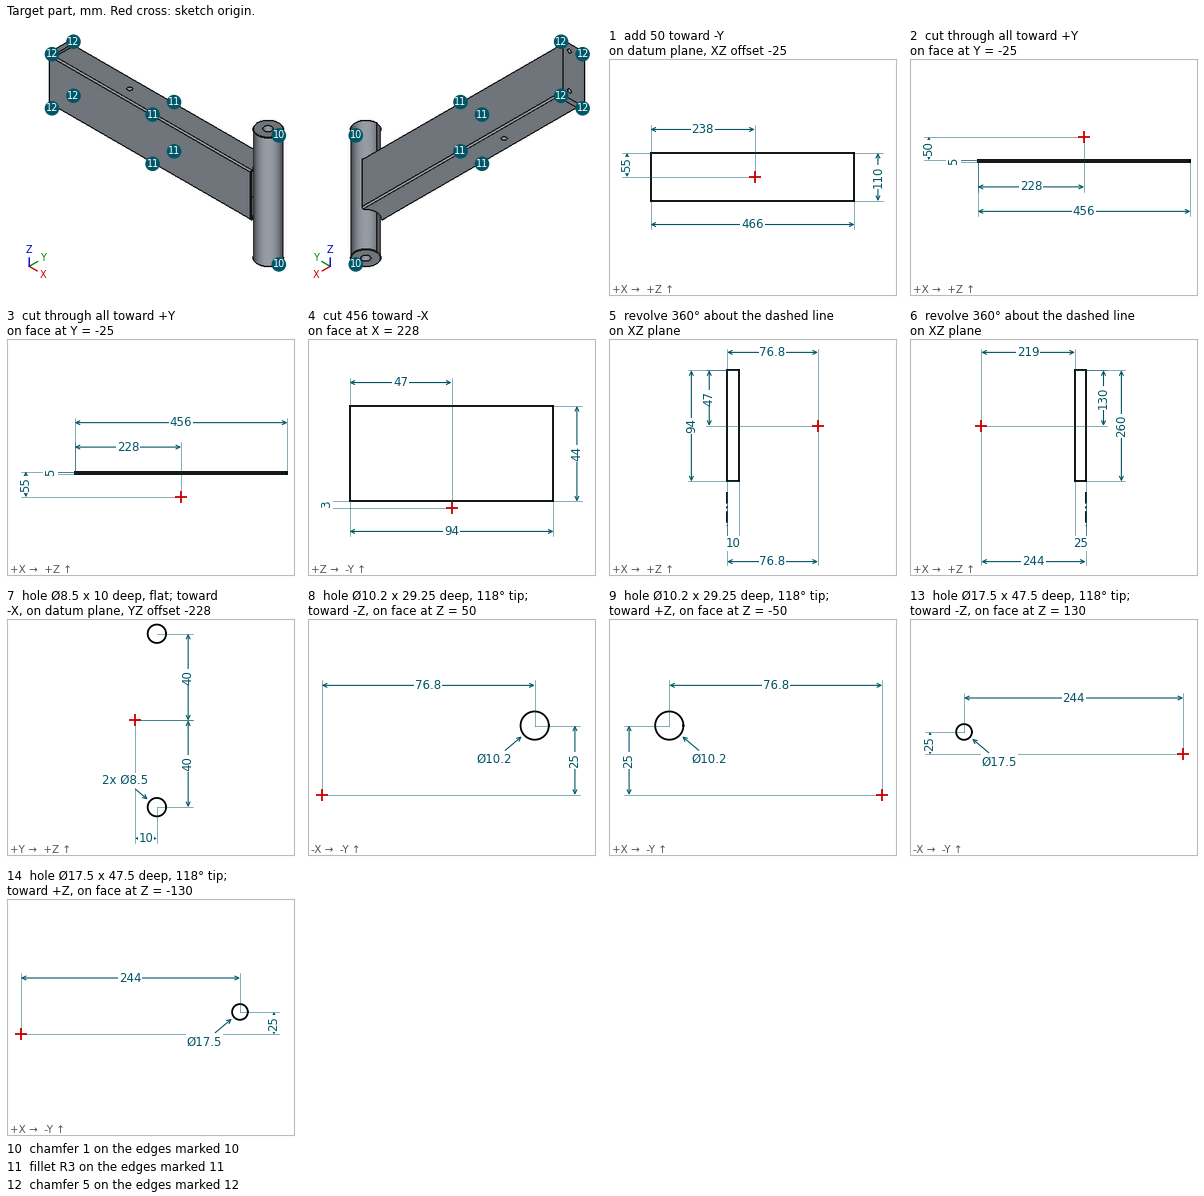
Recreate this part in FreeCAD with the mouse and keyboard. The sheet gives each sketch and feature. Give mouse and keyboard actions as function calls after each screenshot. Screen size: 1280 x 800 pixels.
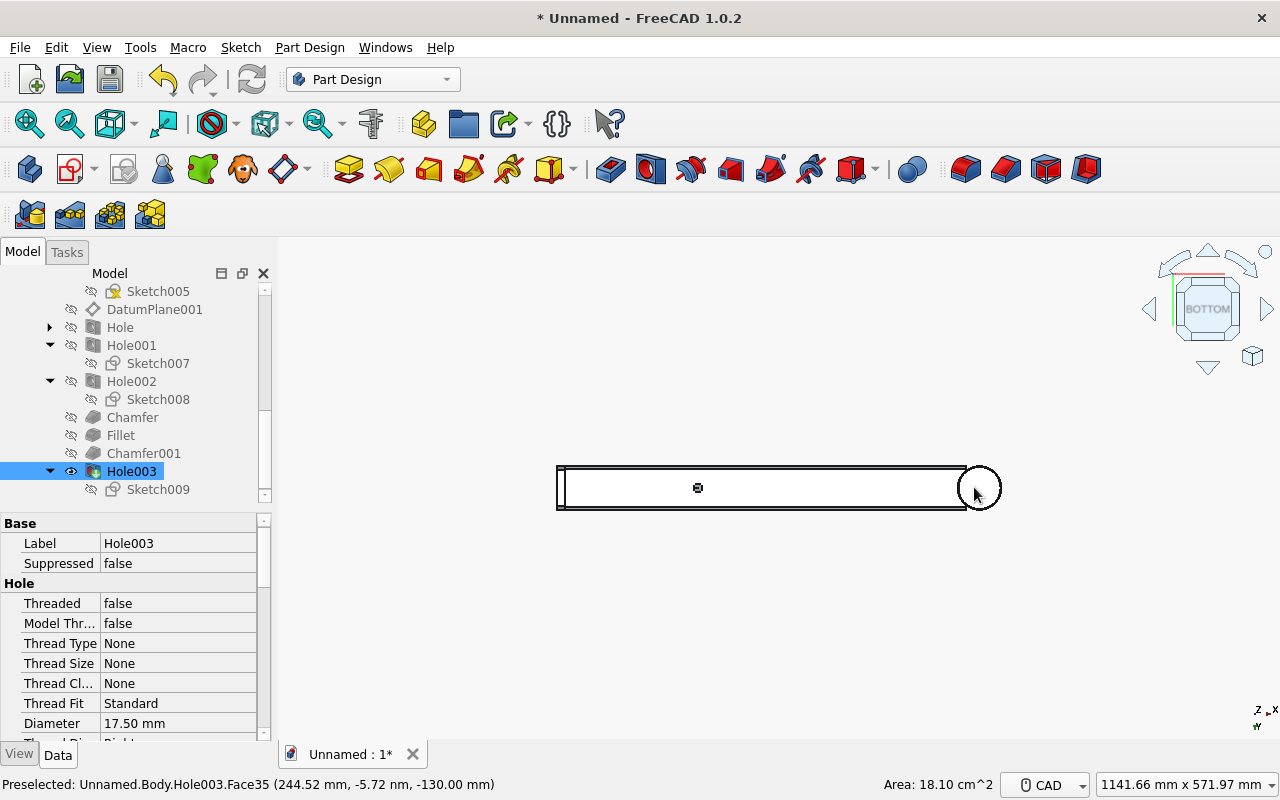
click(70, 170)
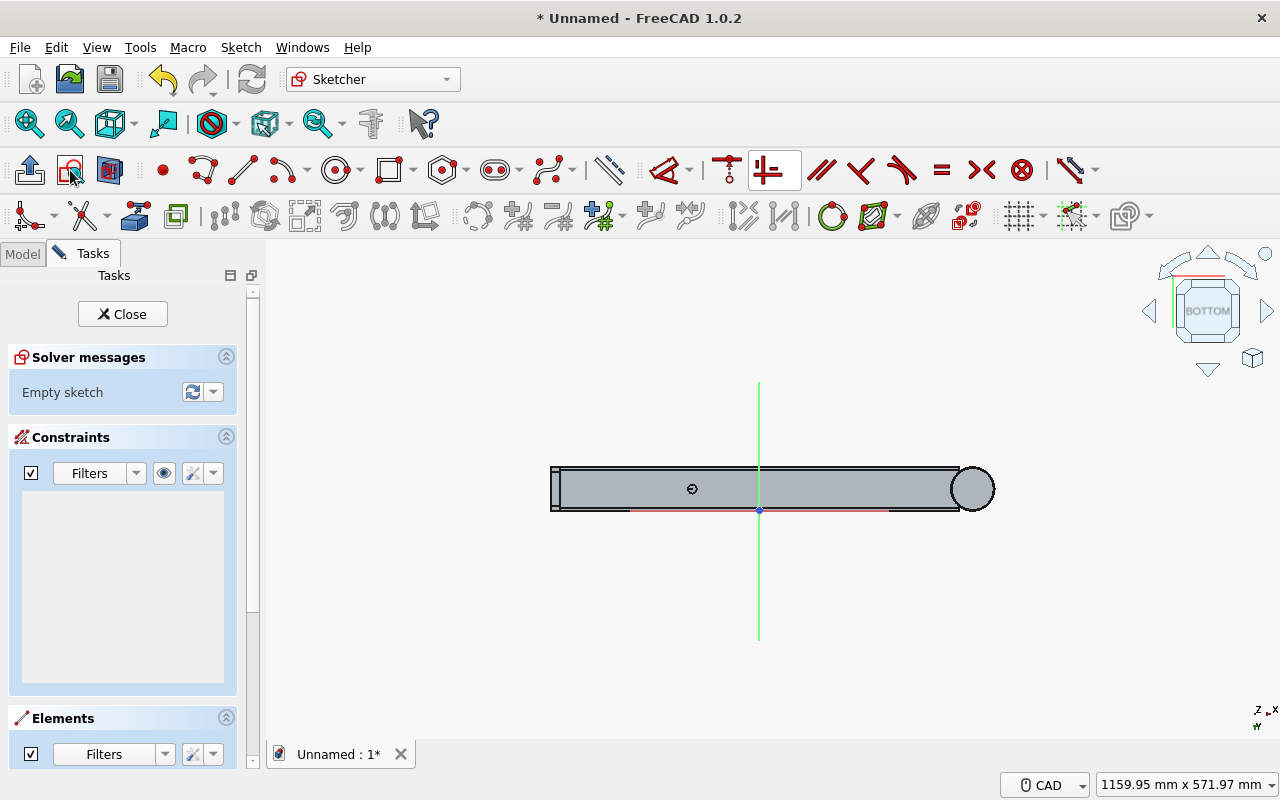
scroll(987, 489, up, 15)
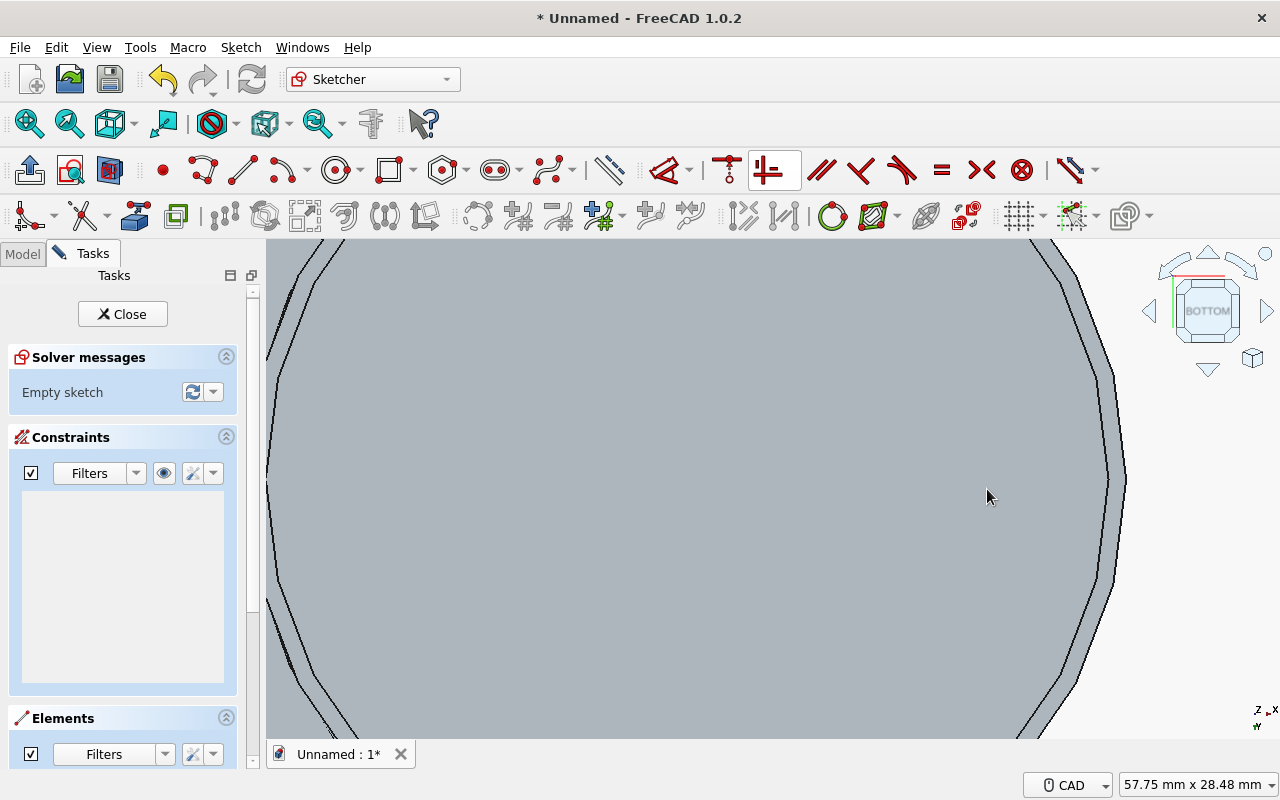
click(336, 170)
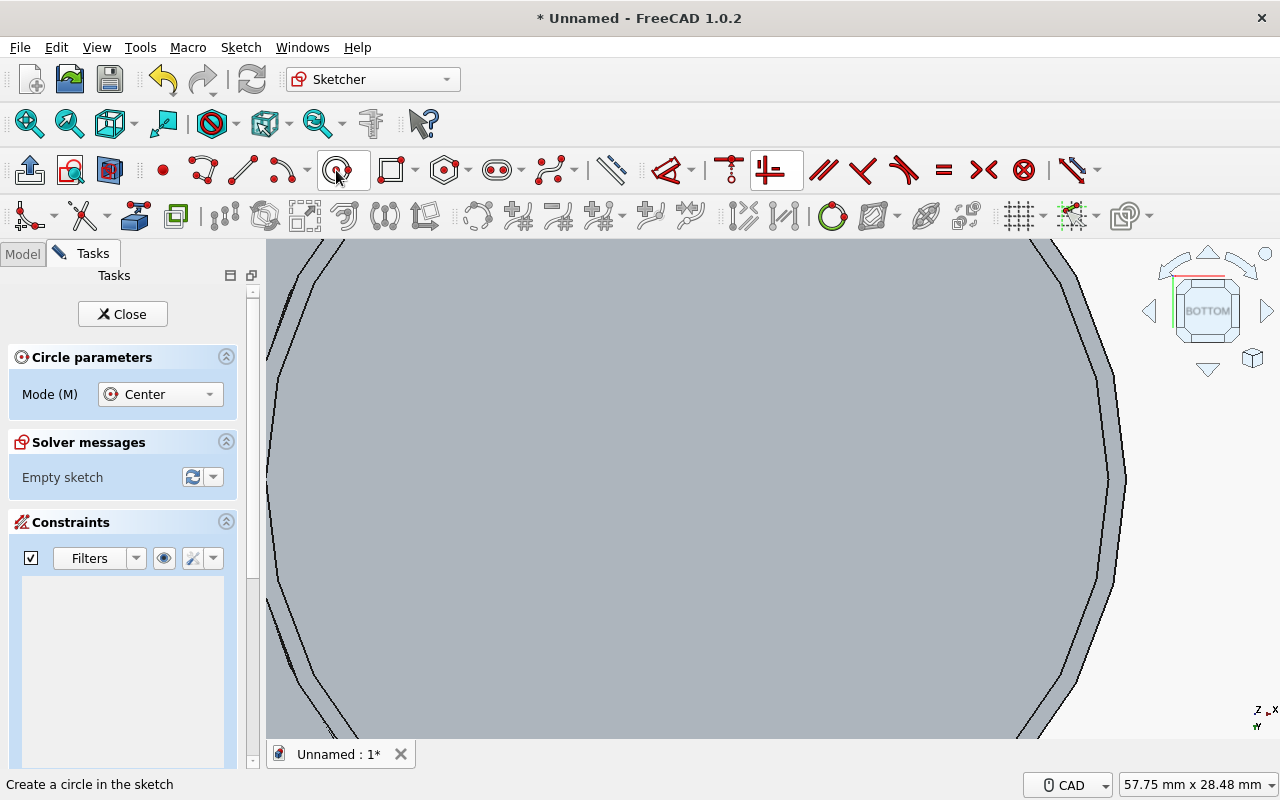
click(687, 479)
move(796, 371)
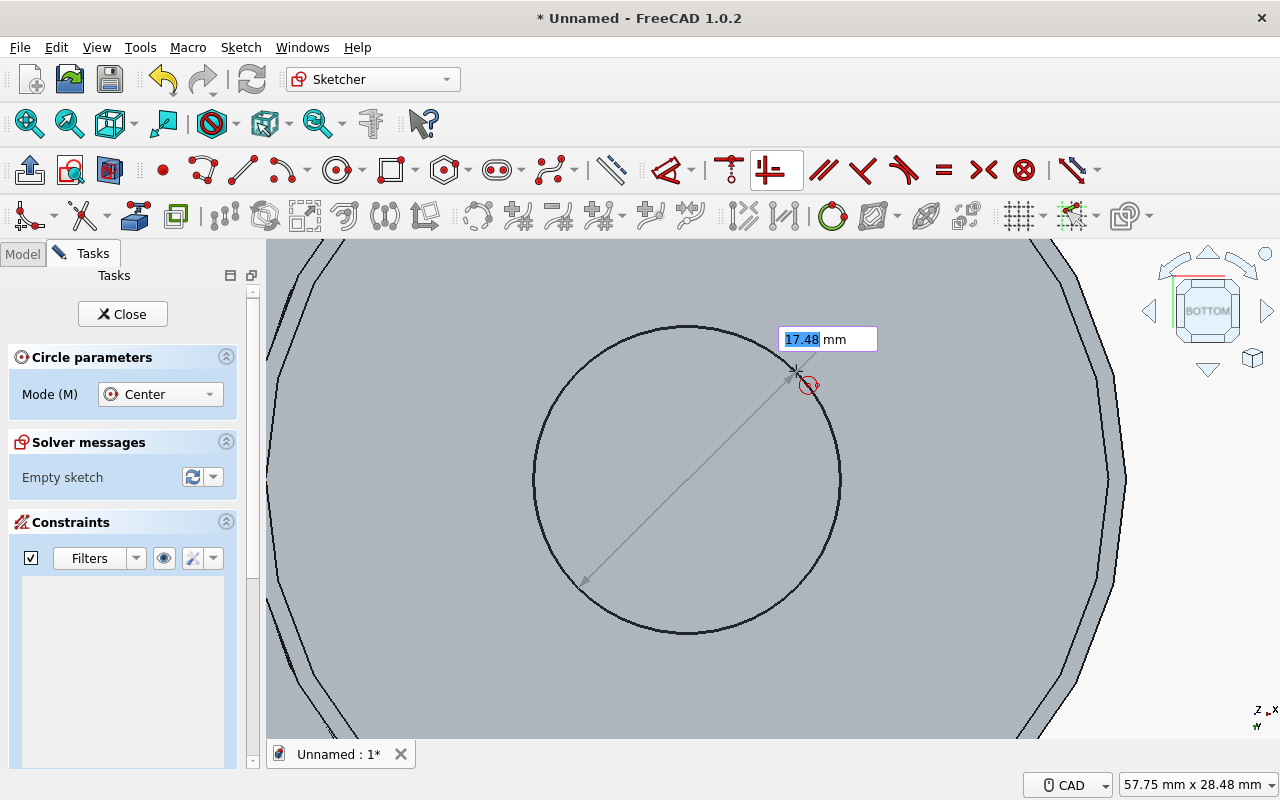
text(17.5)
key(Return)
key(Escape)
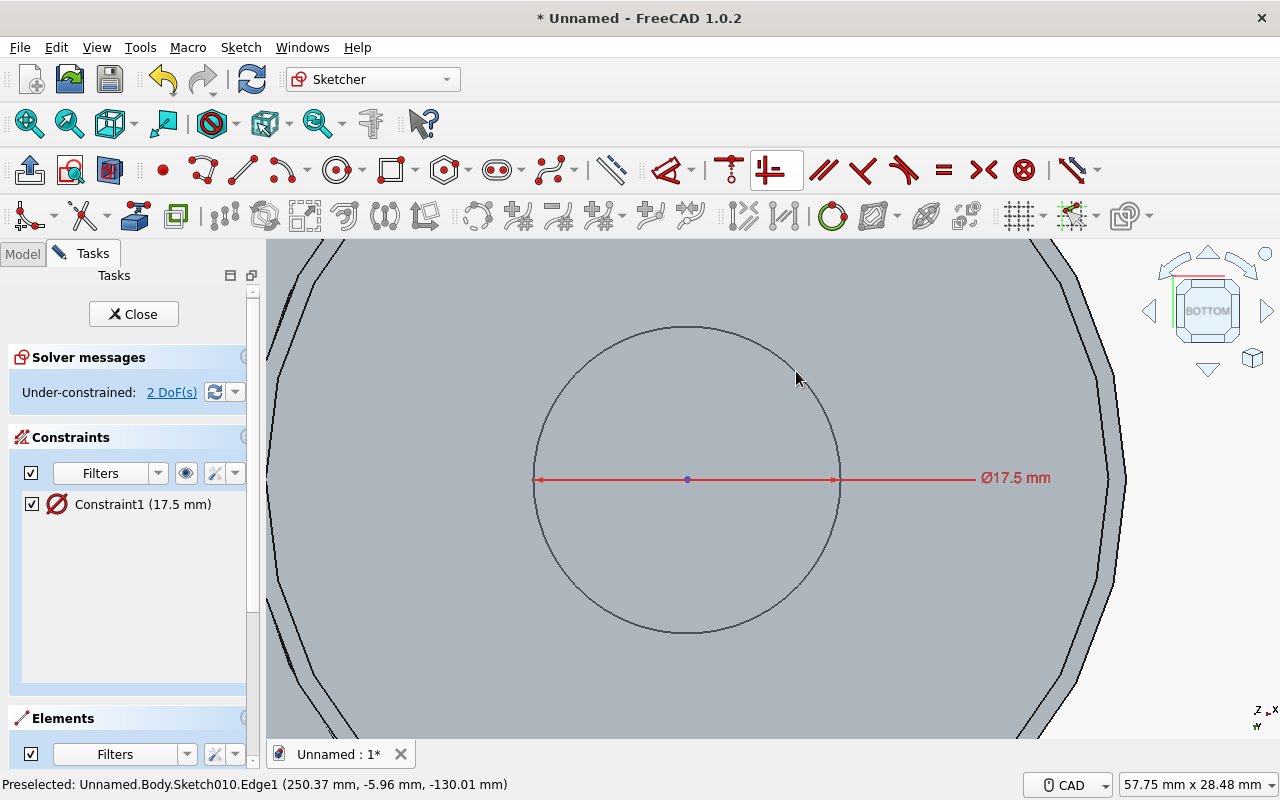
click(666, 170)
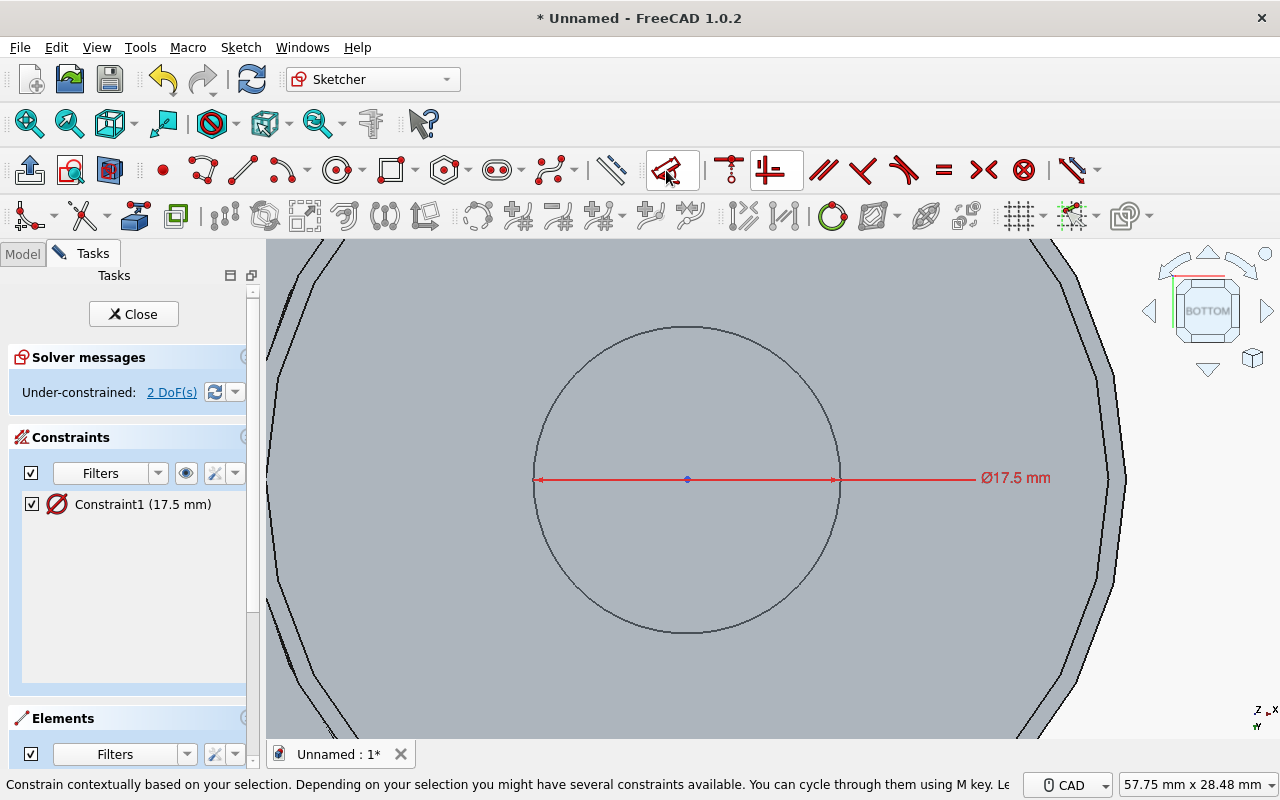
click(687, 480)
click(721, 596)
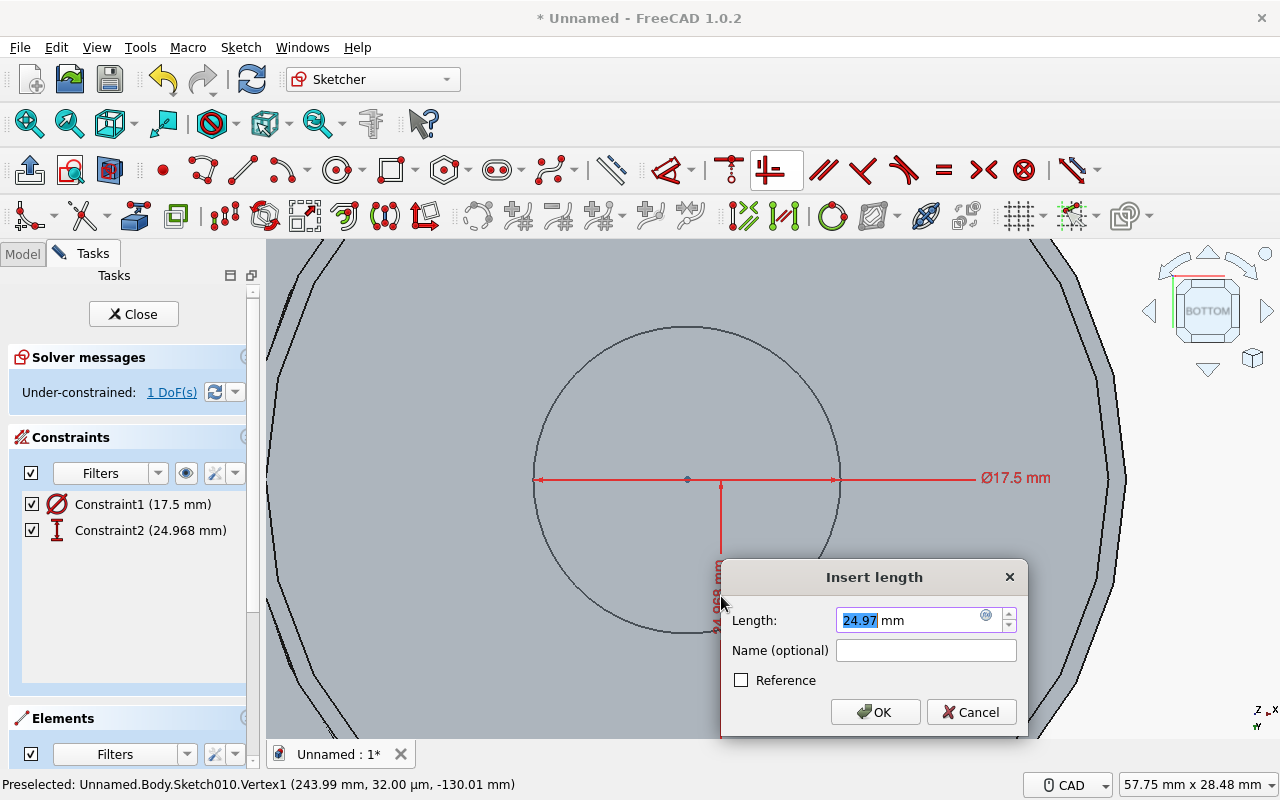
text(25)
key(Return)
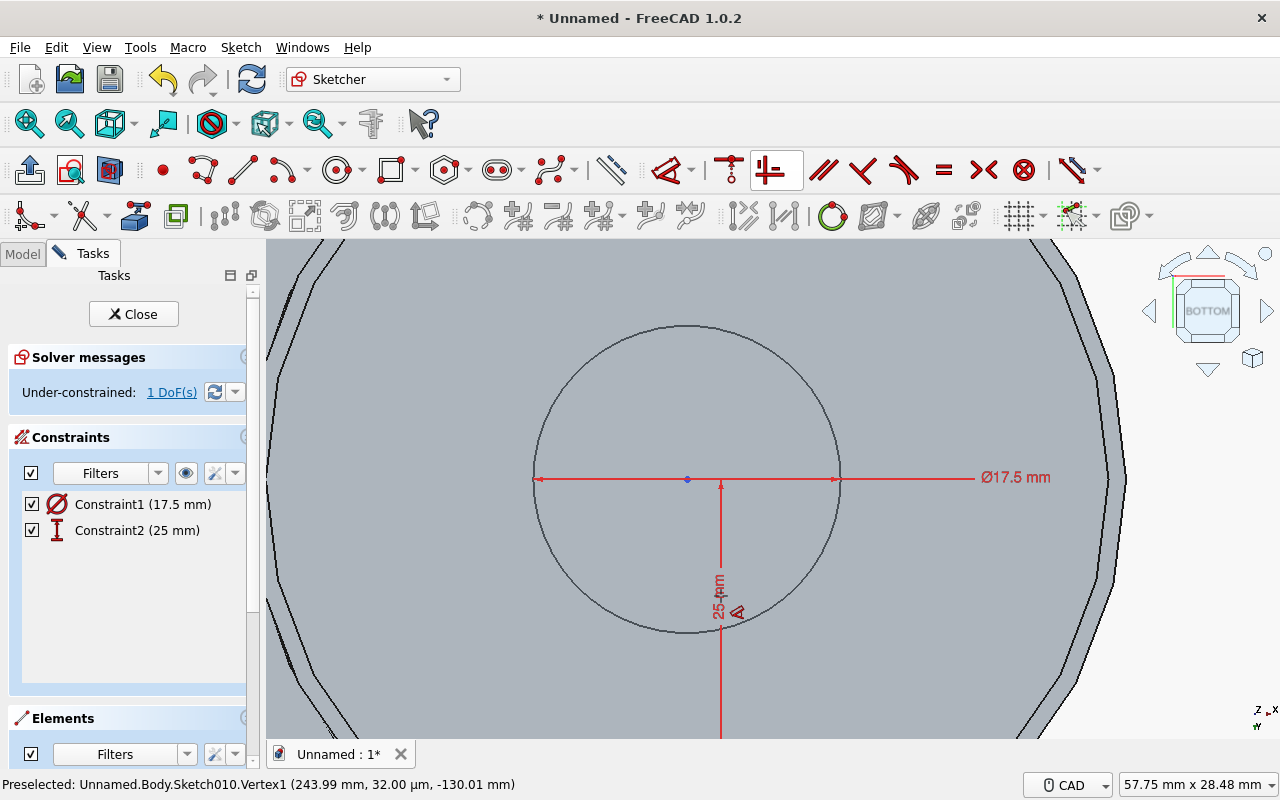
click(687, 479)
click(490, 445)